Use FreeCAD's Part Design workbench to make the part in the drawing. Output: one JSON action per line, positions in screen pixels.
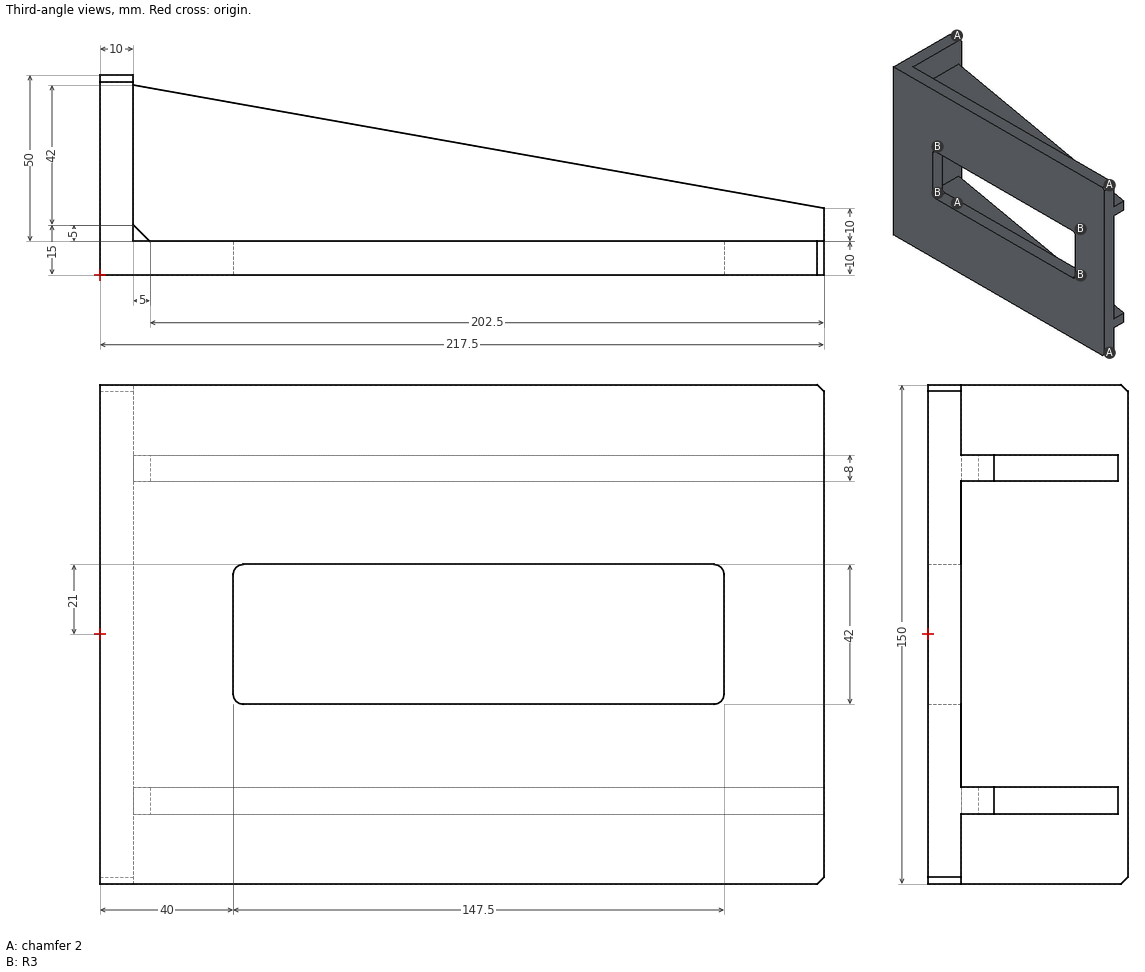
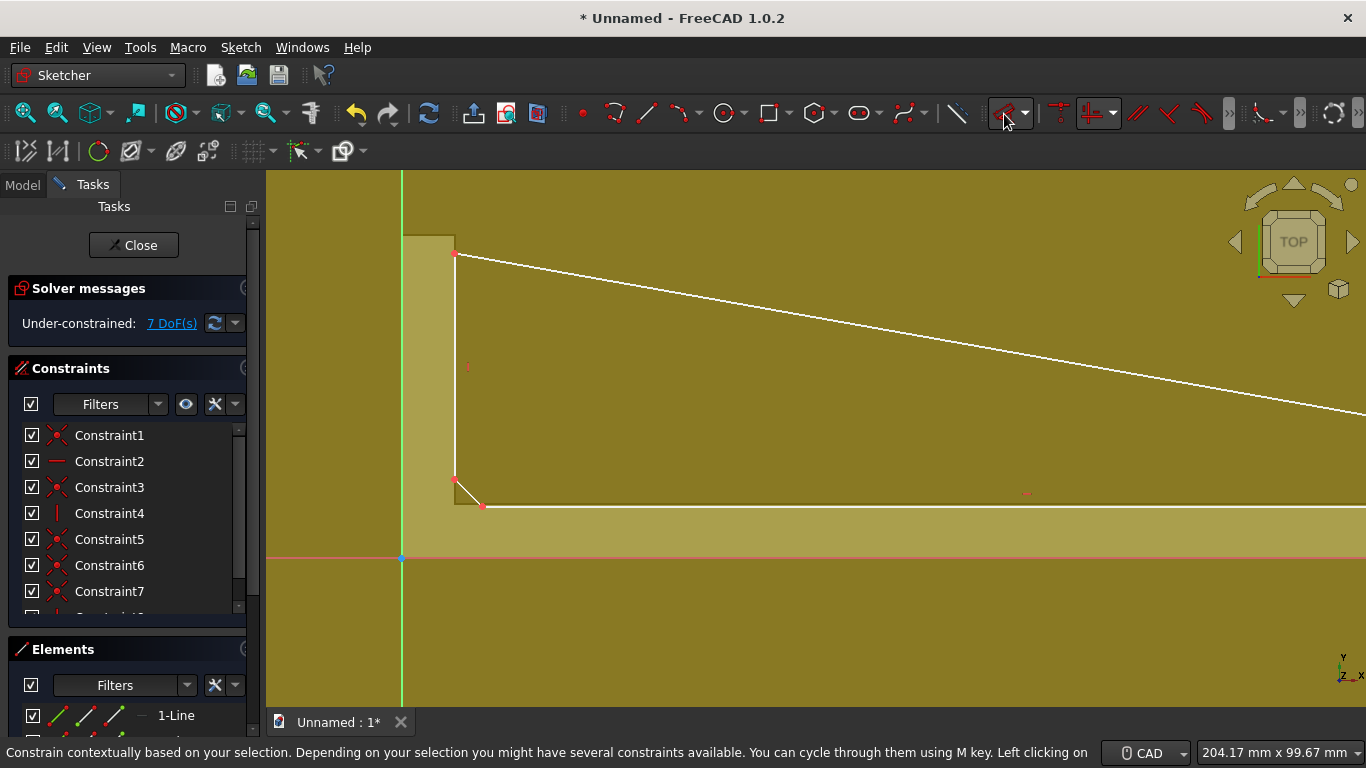
{"action": "scroll", "coordinate": [456, 480], "scroll_direction": "down", "scroll_amount": 3}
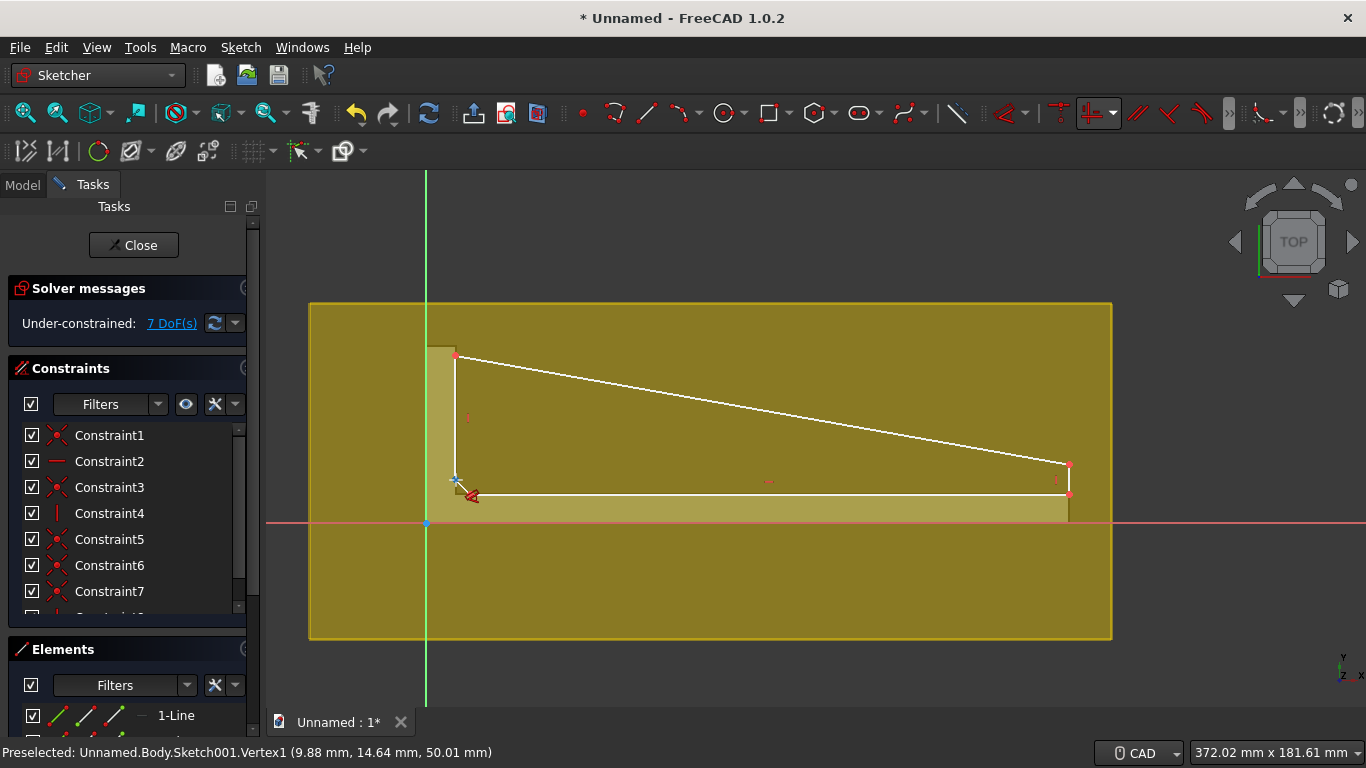
{"action": "scroll", "coordinate": [1069, 486], "scroll_direction": "up", "scroll_amount": 3}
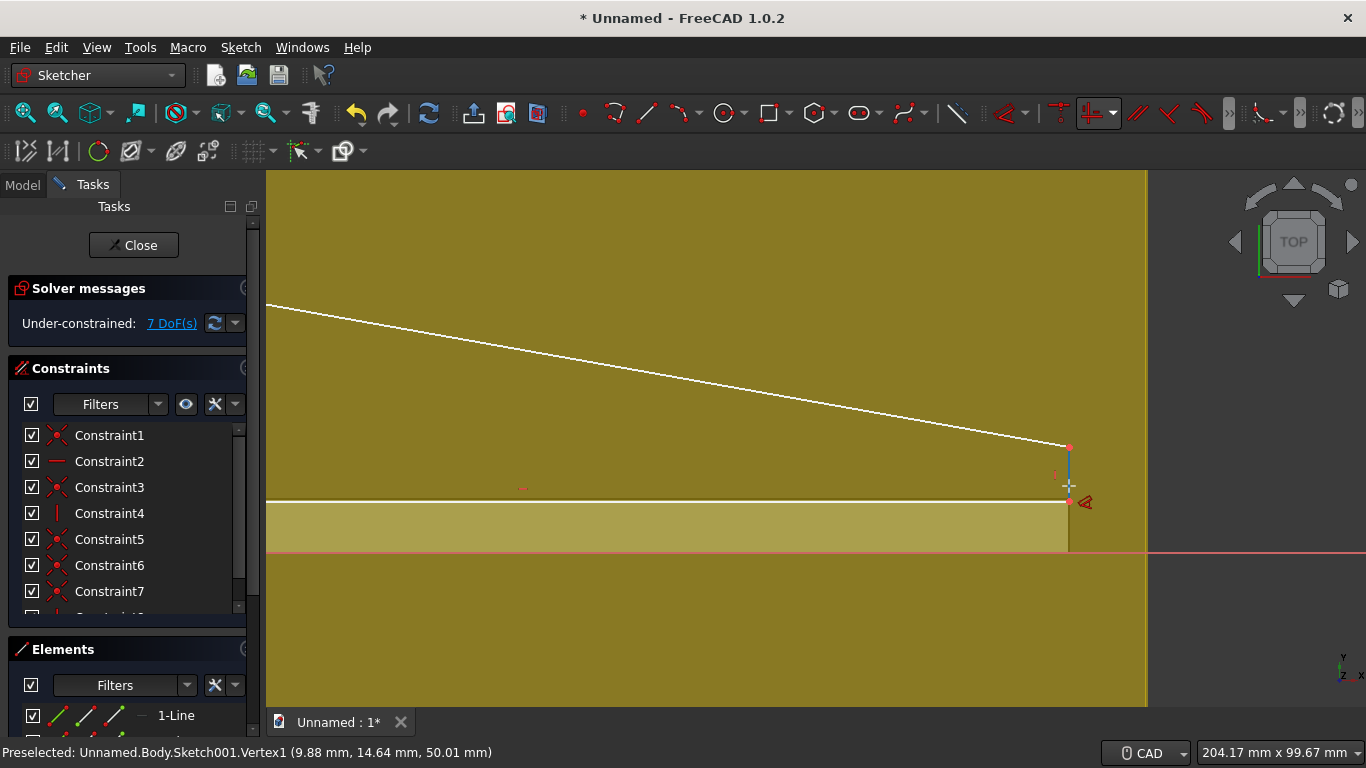
{"action": "left_click", "coordinate": [1069, 485]}
{"action": "left_click", "coordinate": [1103, 474]}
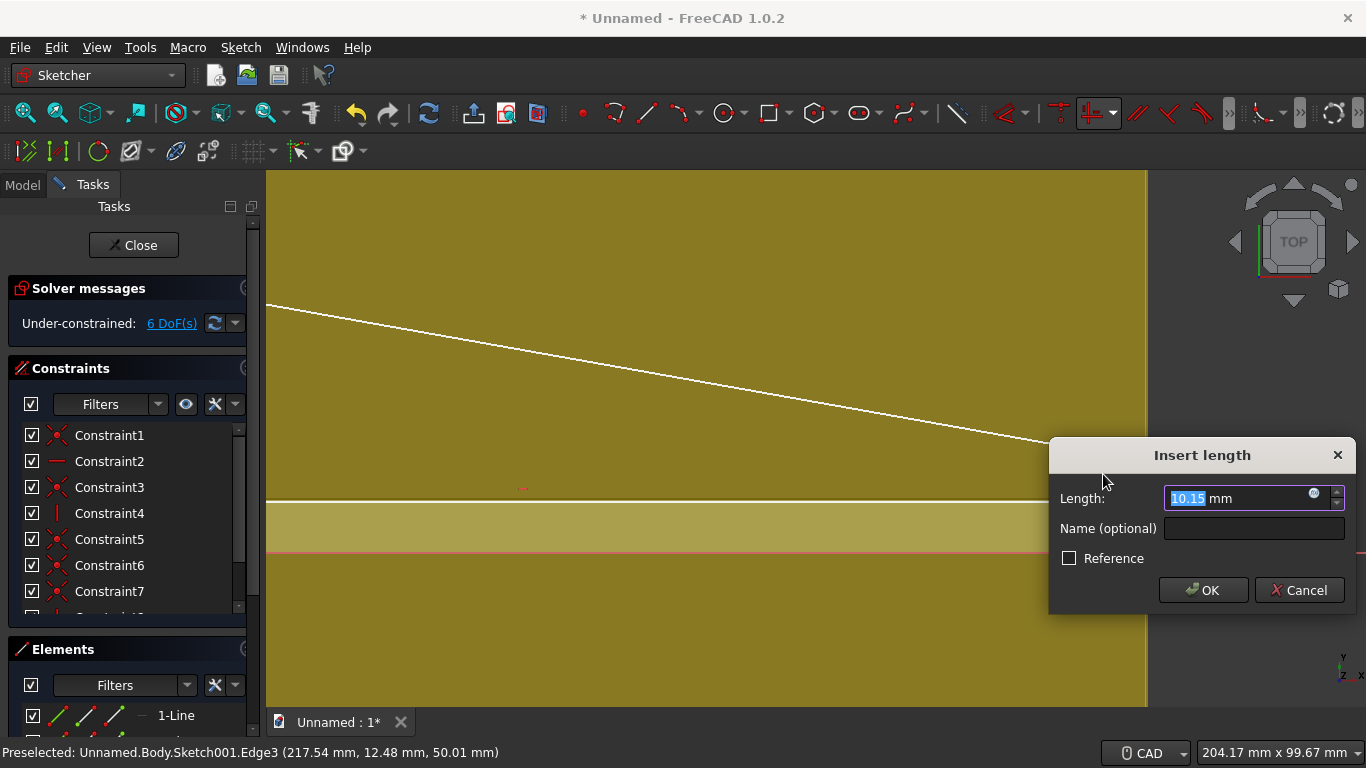
{"action": "type", "text": "10"}
{"action": "key", "text": "Return"}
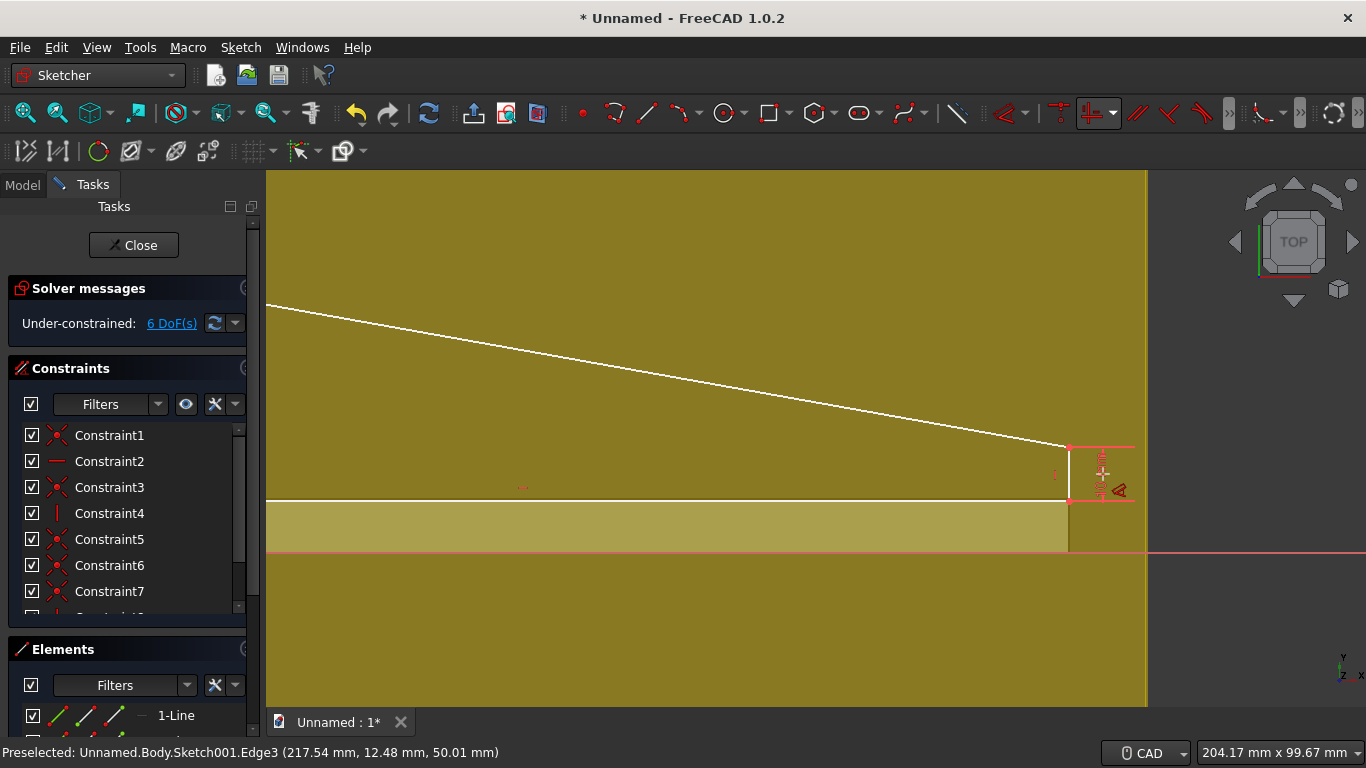
{"action": "scroll", "coordinate": [1069, 486], "scroll_direction": "down", "scroll_amount": 3}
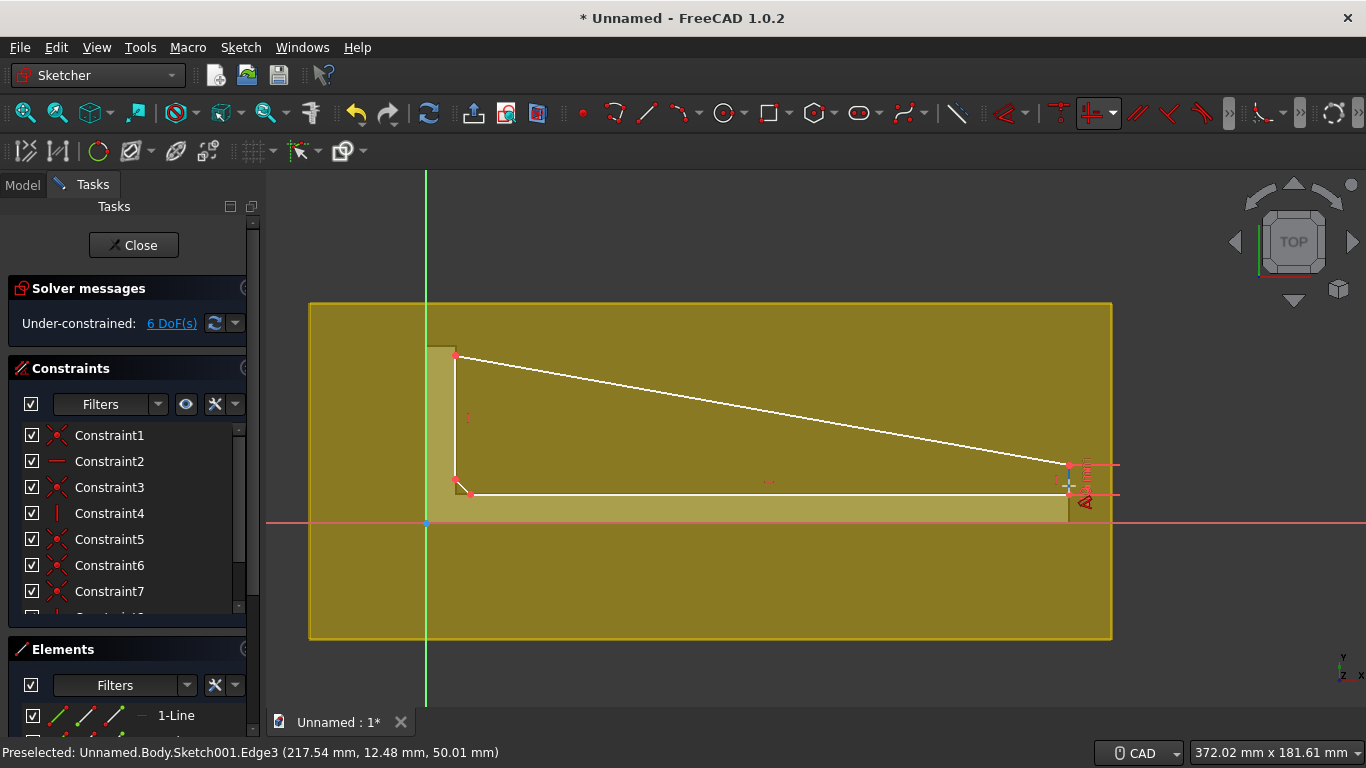
{"action": "left_click", "coordinate": [455, 393]}
{"action": "left_click", "coordinate": [489, 418]}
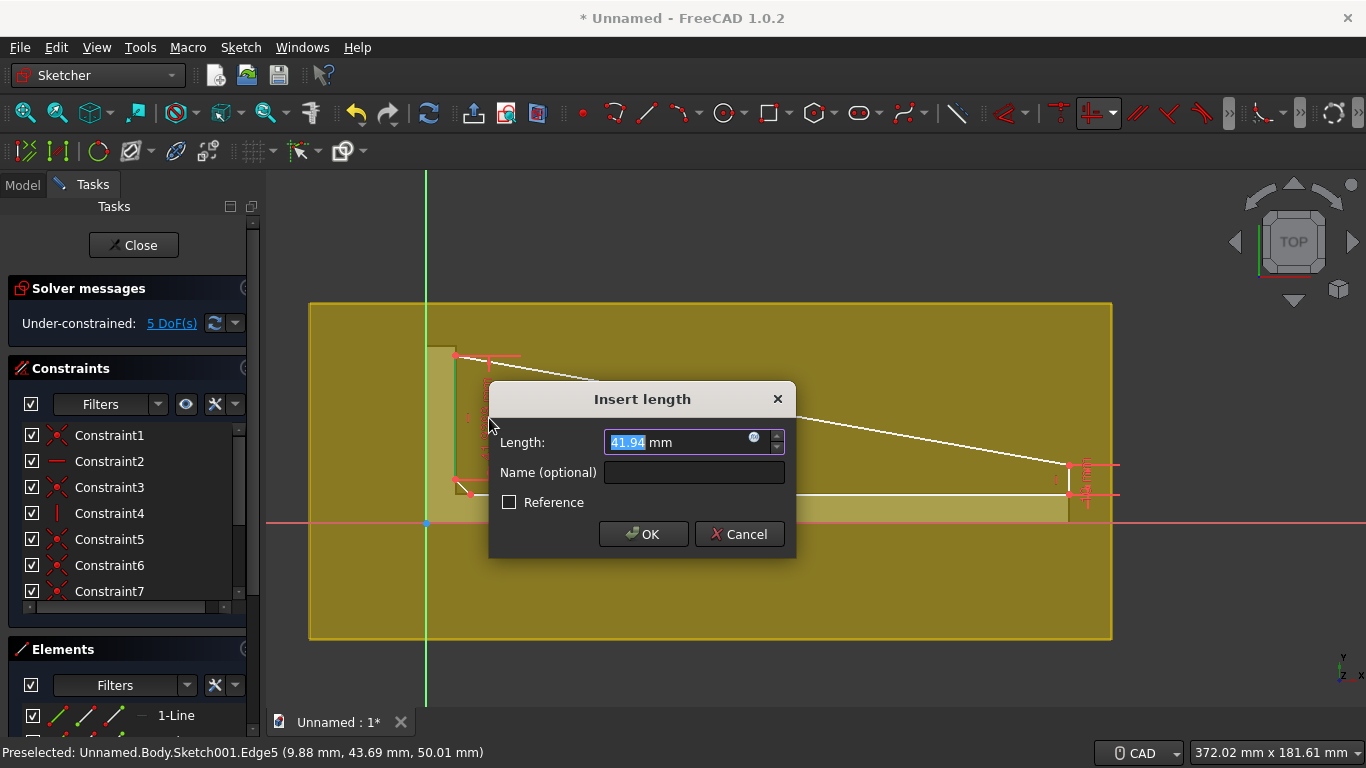
{"action": "type", "text": "42"}
{"action": "key", "text": "Return"}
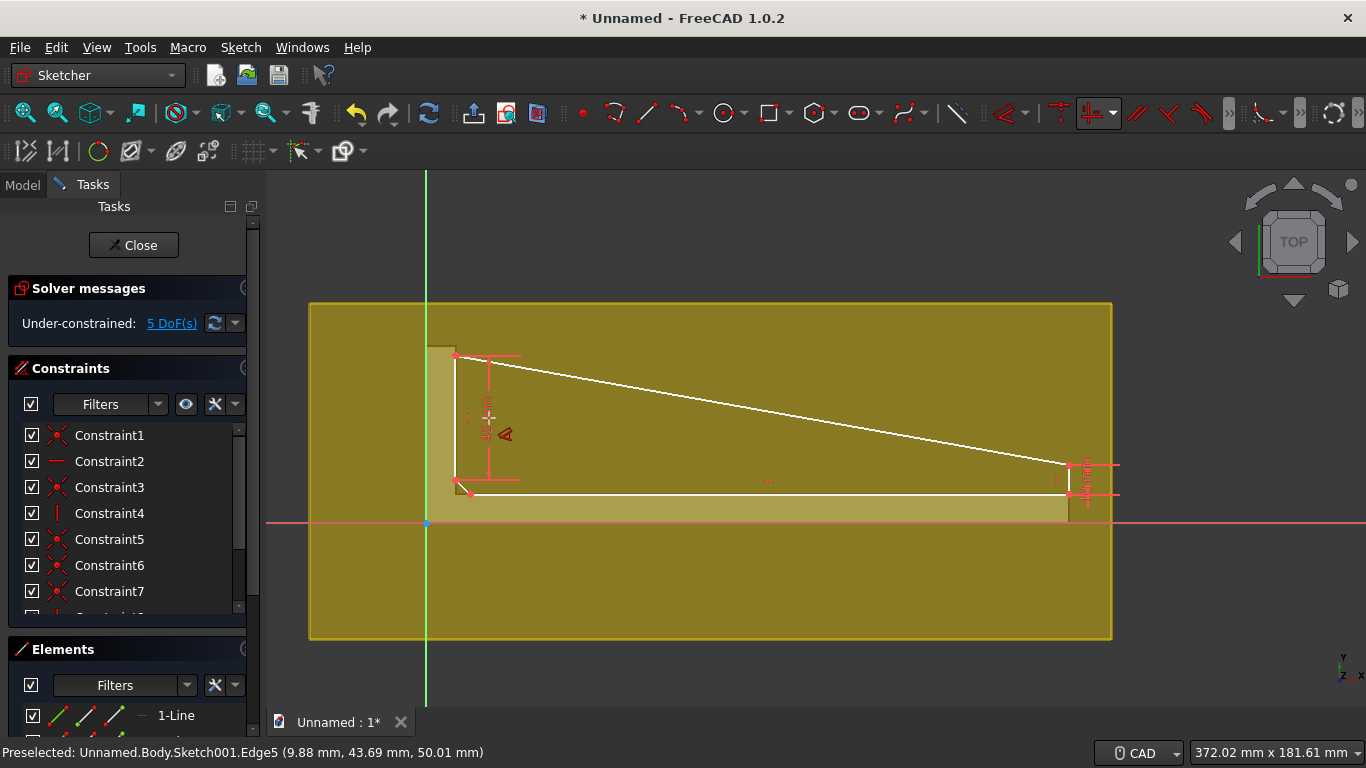
{"action": "scroll", "coordinate": [463, 487], "scroll_direction": "up", "scroll_amount": 5}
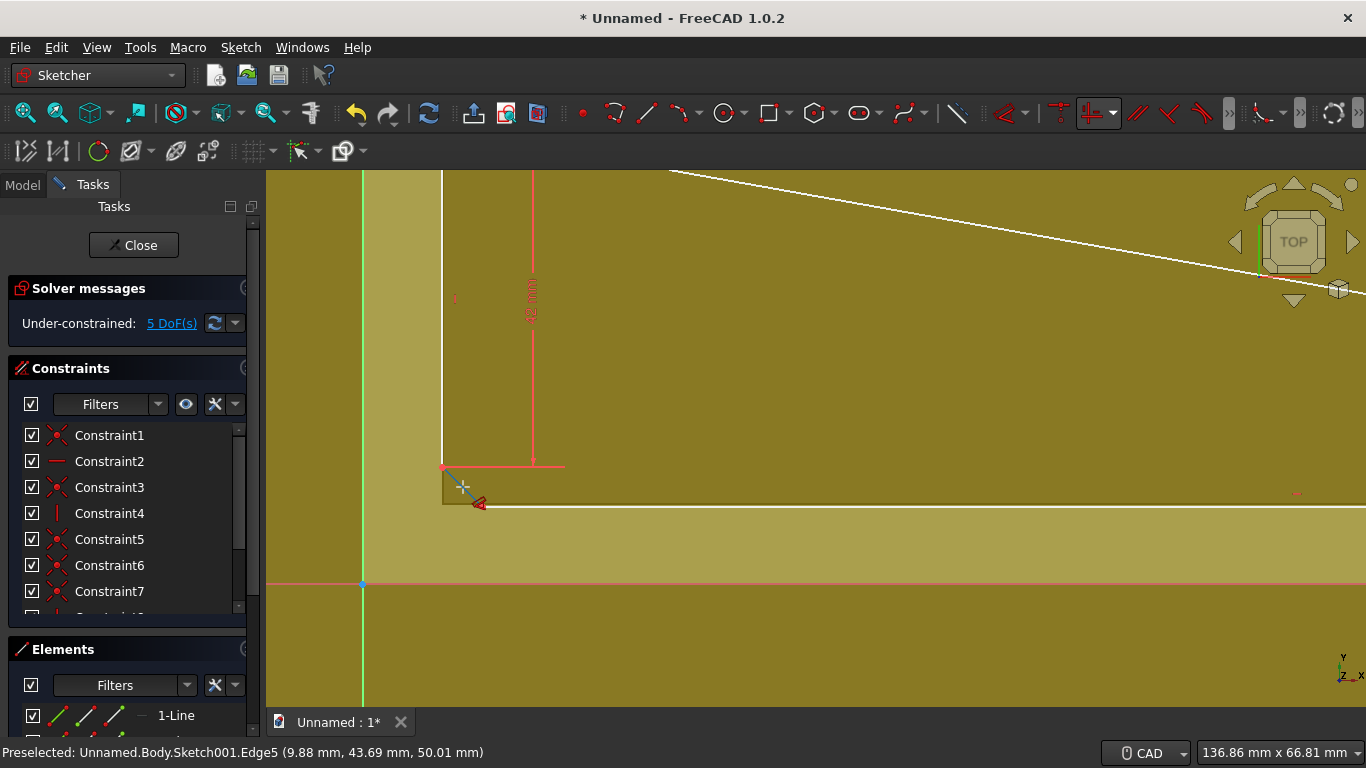
{"action": "left_click", "coordinate": [463, 487]}
{"action": "left_click", "coordinate": [463, 541]}